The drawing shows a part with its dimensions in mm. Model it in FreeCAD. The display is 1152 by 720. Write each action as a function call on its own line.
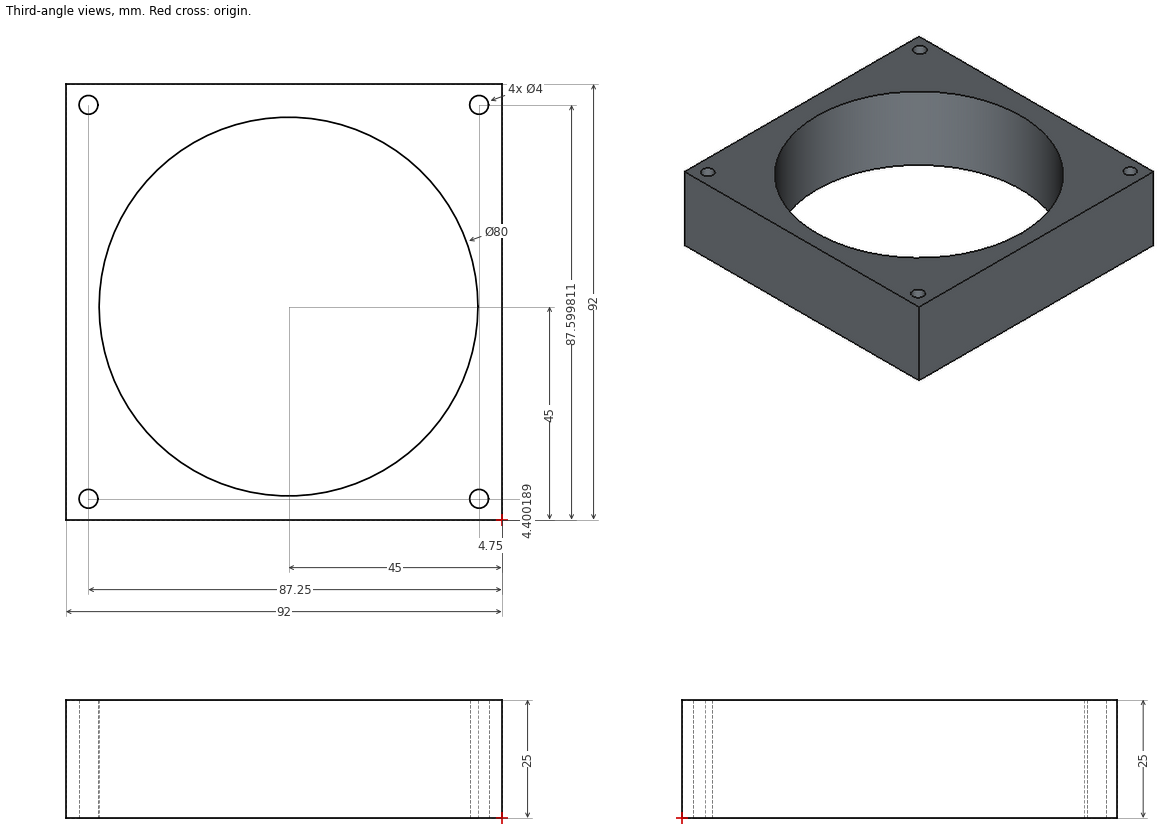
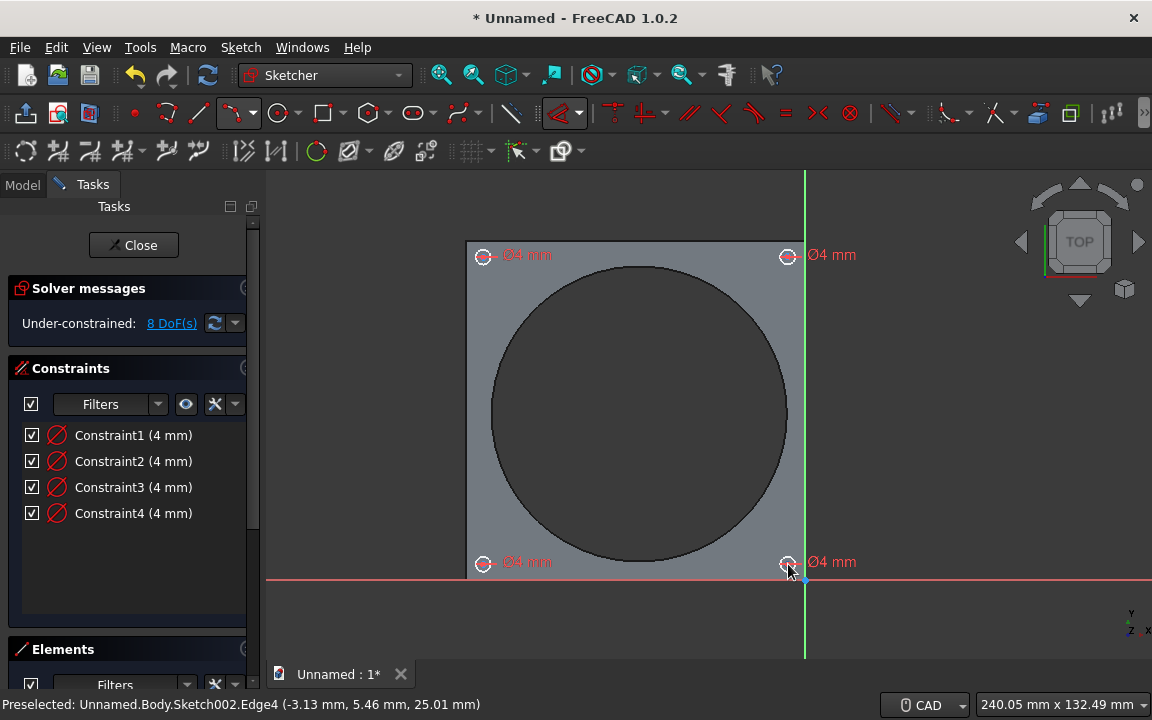
click(788, 257)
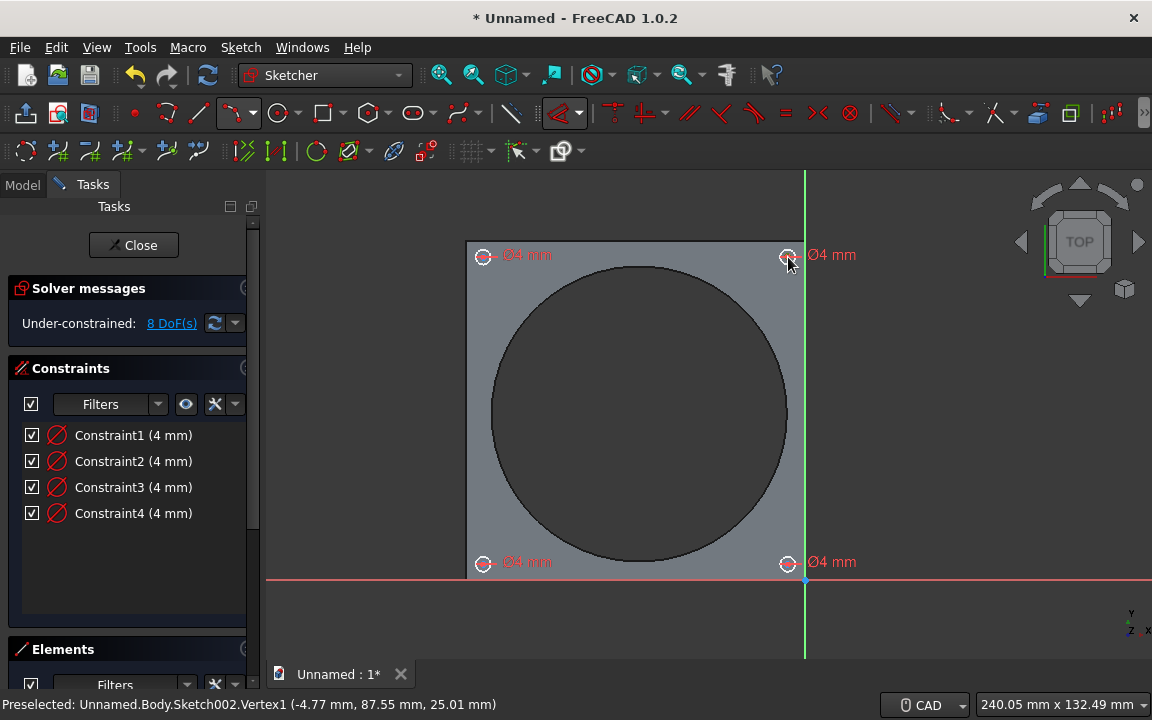
click(483, 257)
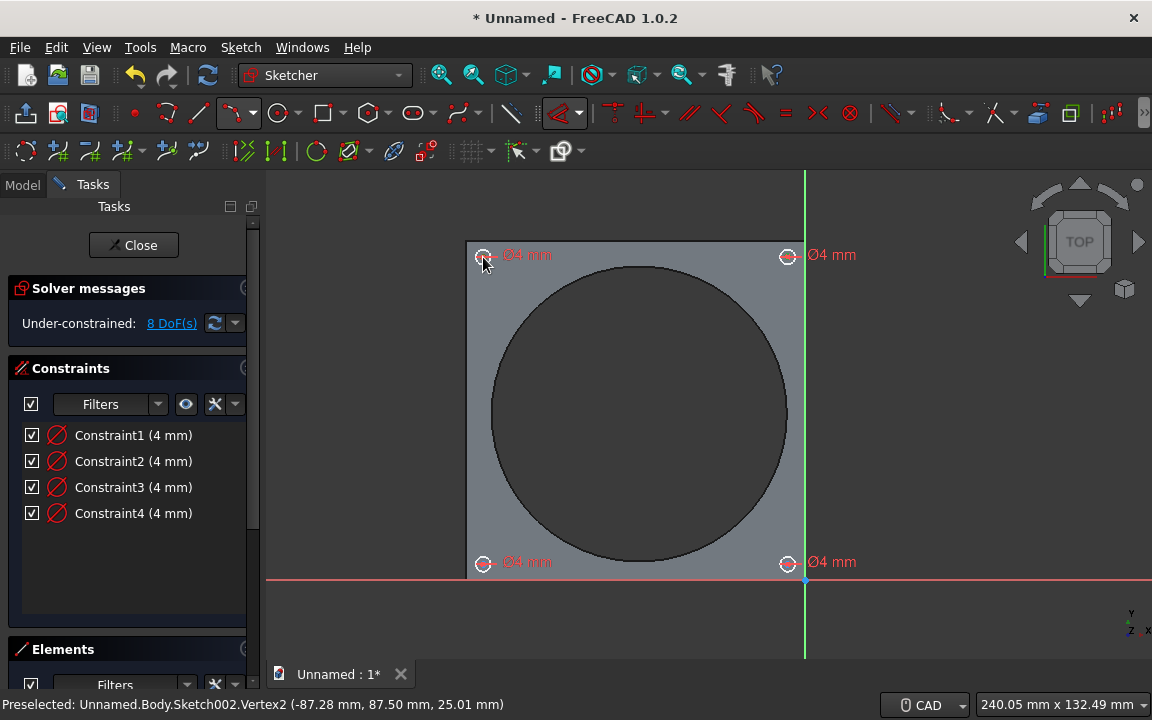
key(h)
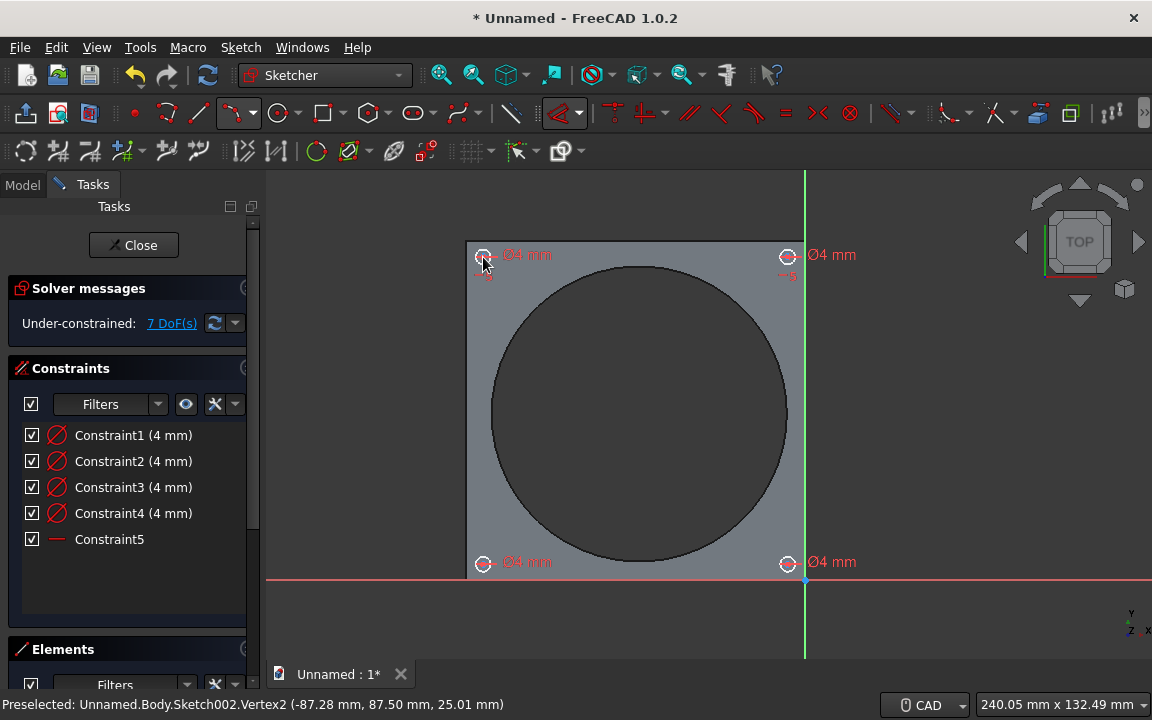
click(483, 257)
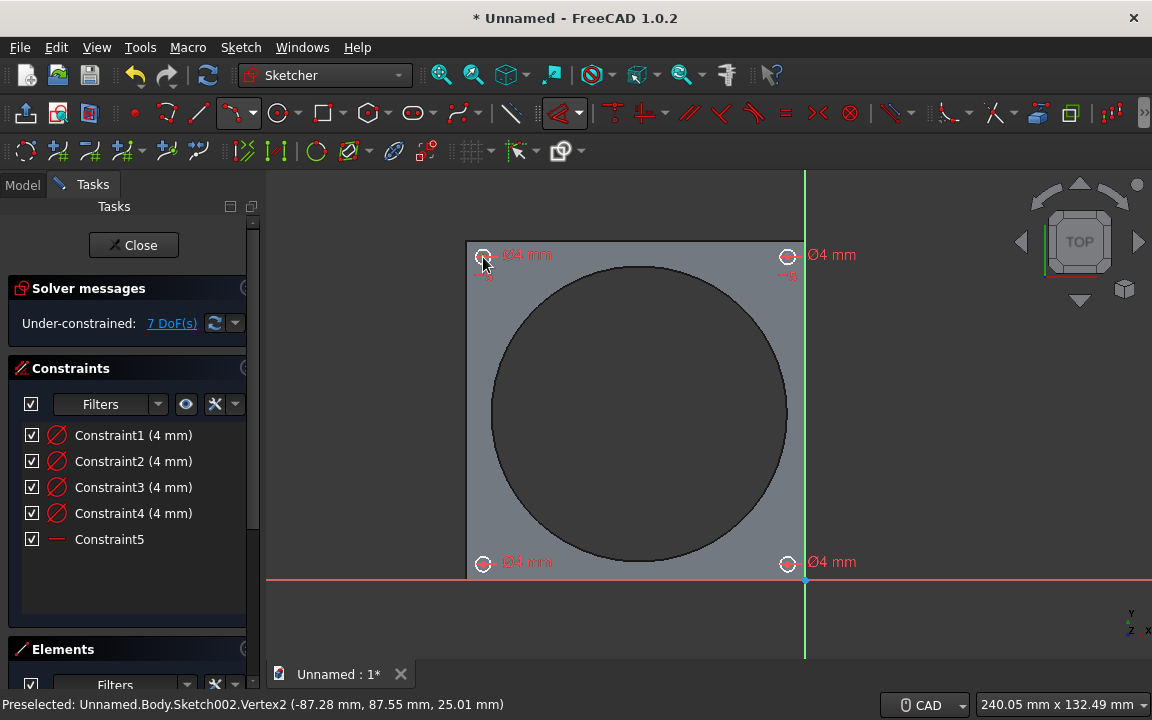
click(483, 564)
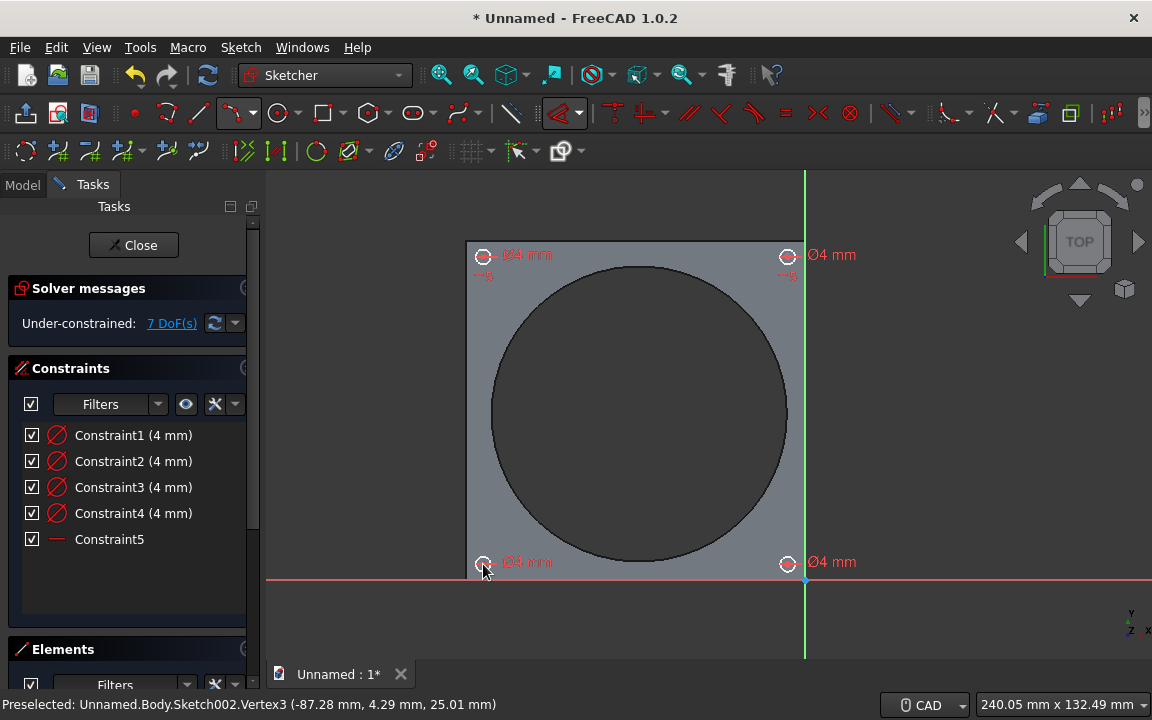
key(v)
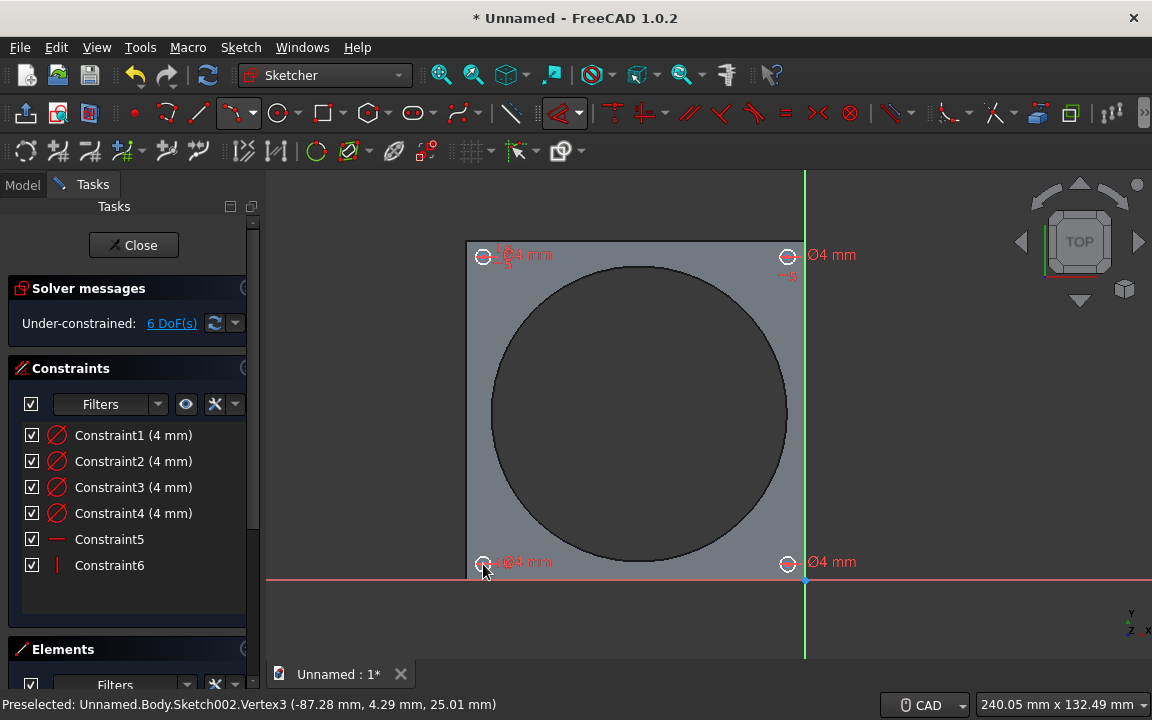
click(788, 257)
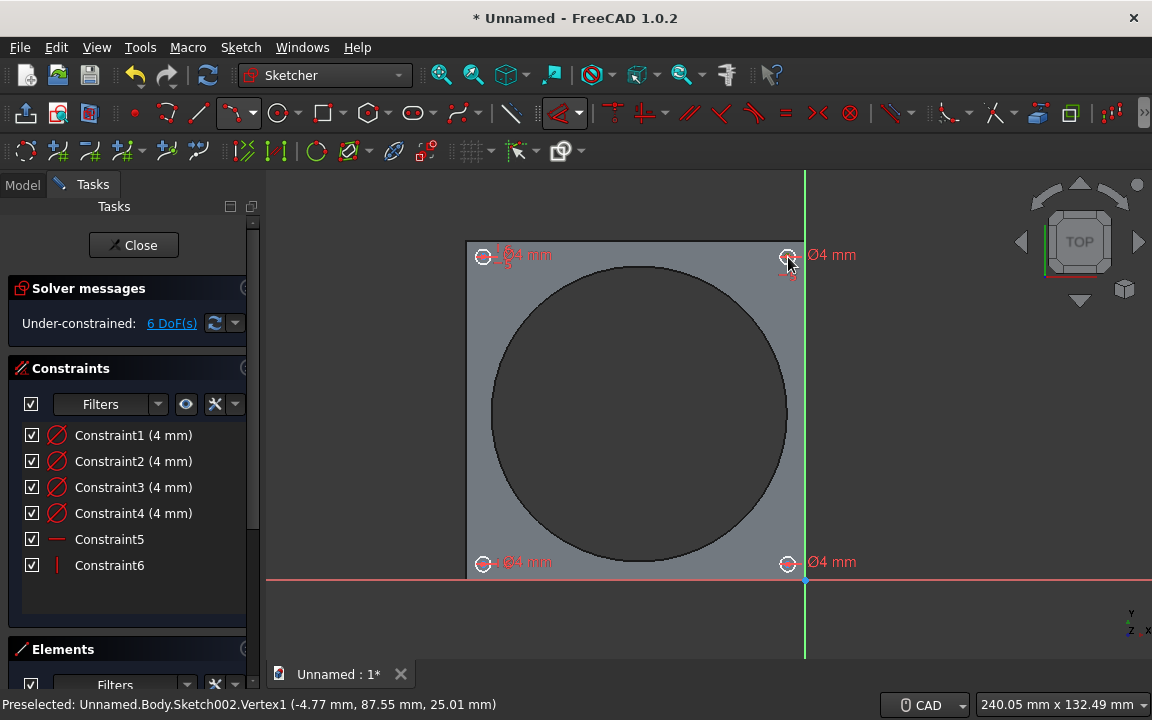
click(788, 564)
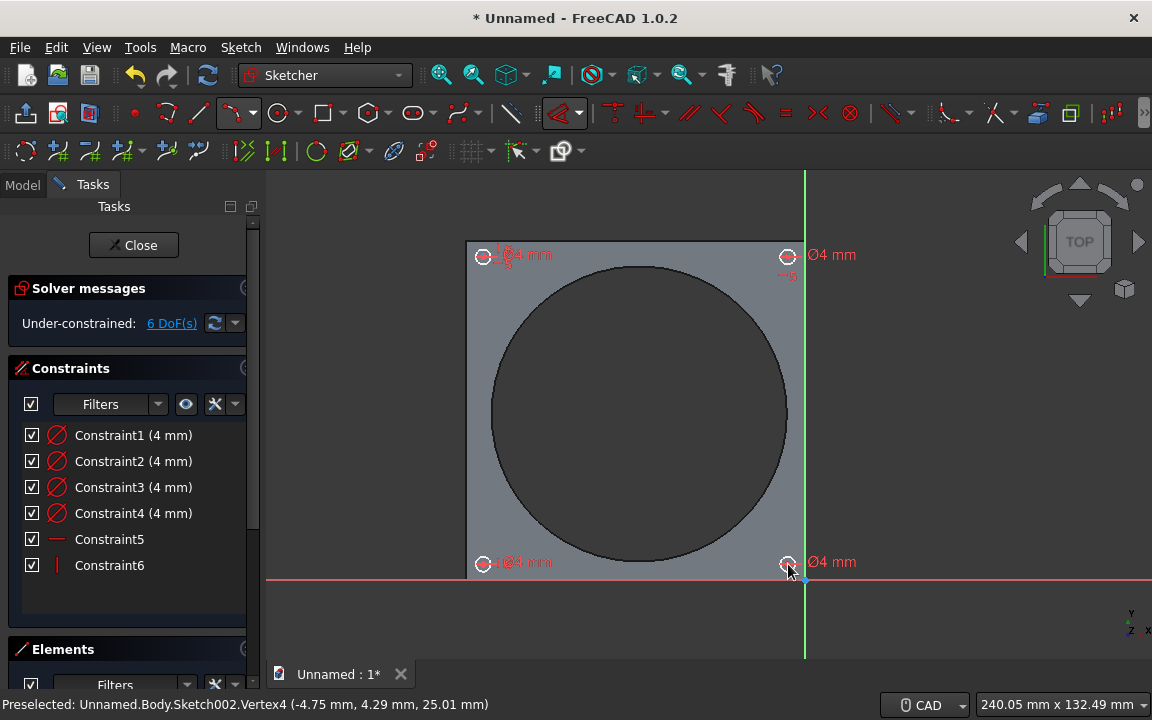
key(v)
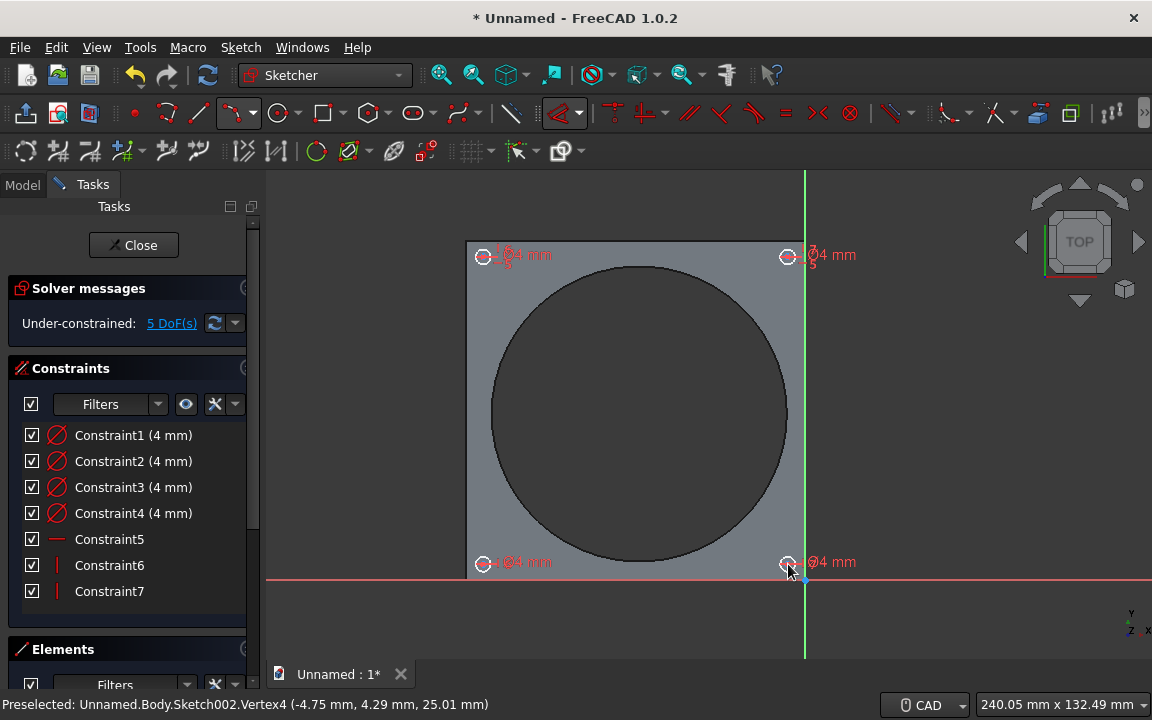
click(483, 564)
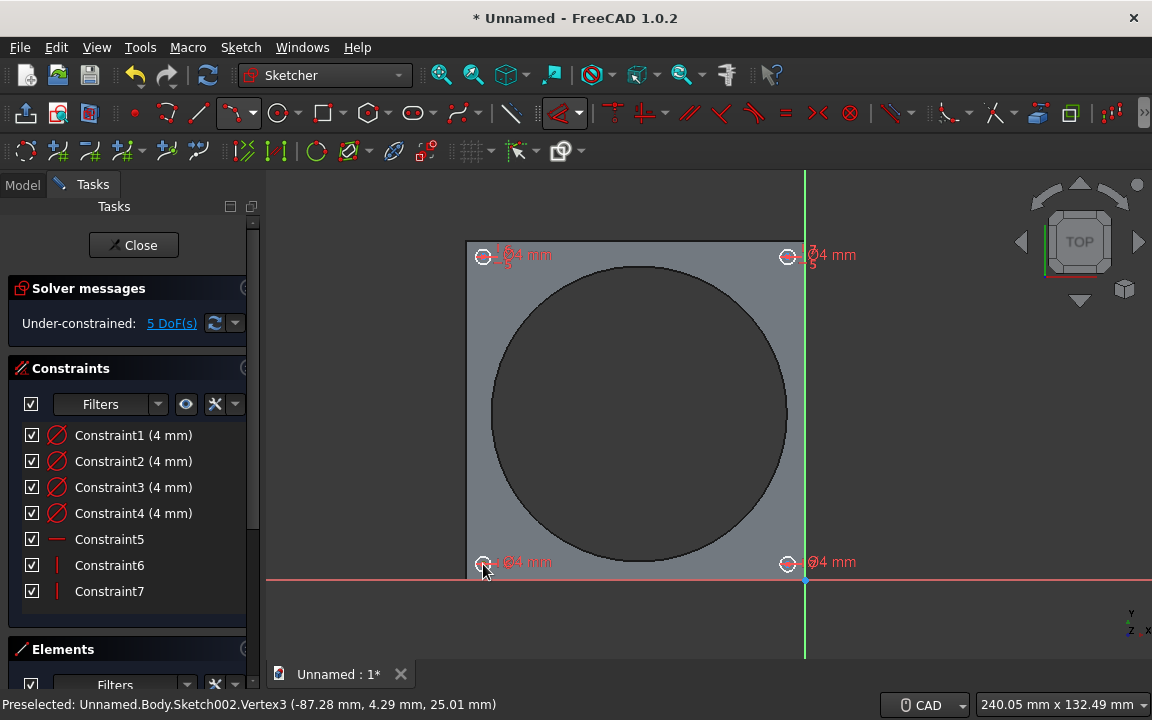
click(788, 564)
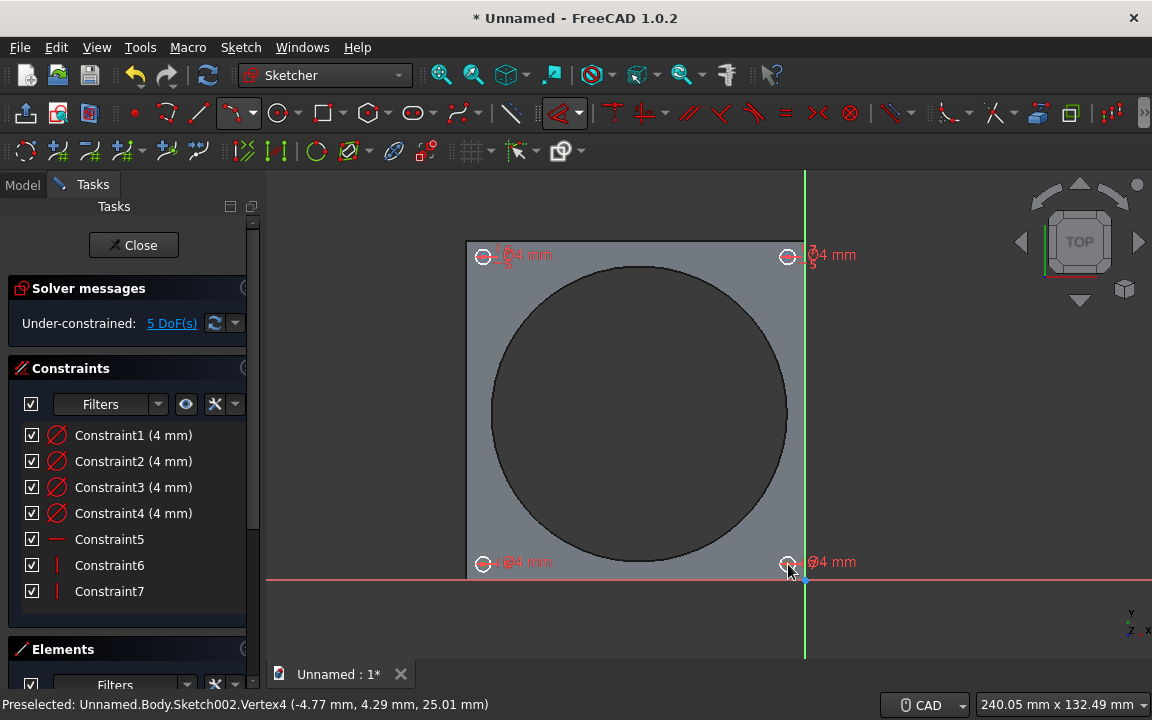
key(h)